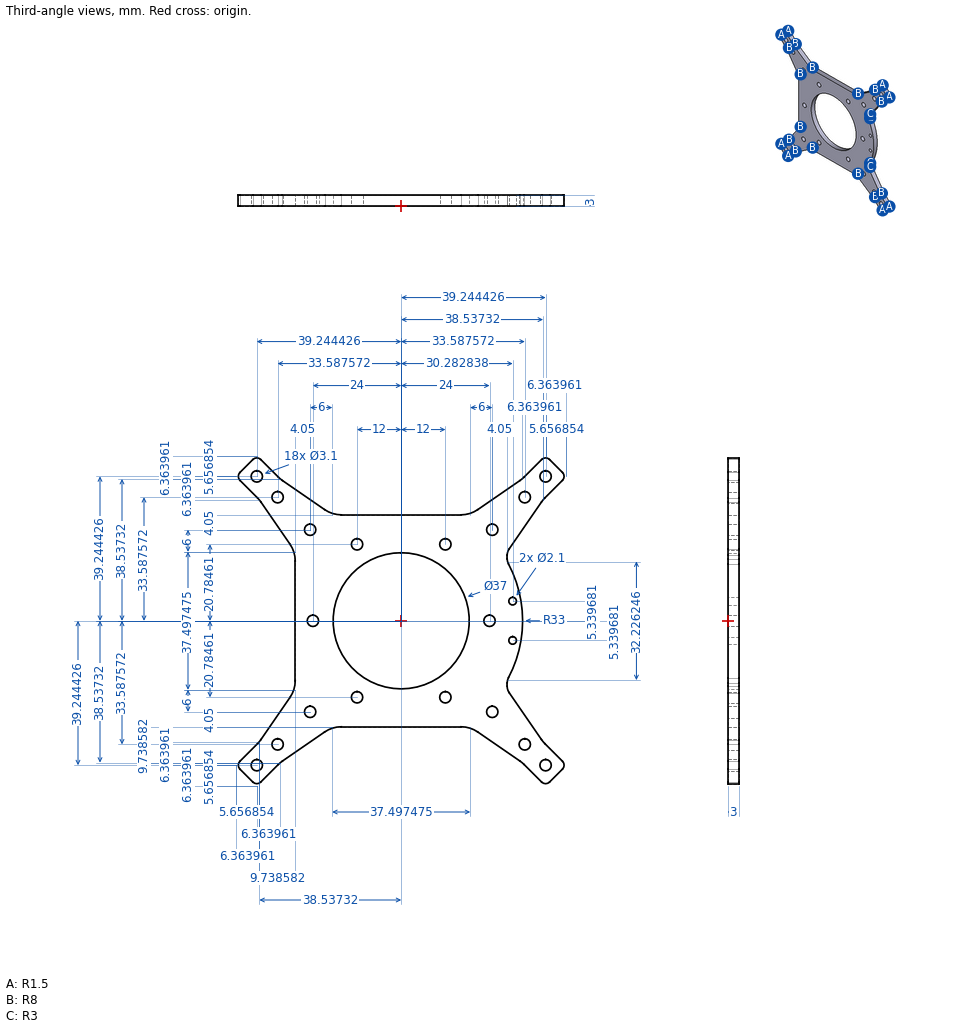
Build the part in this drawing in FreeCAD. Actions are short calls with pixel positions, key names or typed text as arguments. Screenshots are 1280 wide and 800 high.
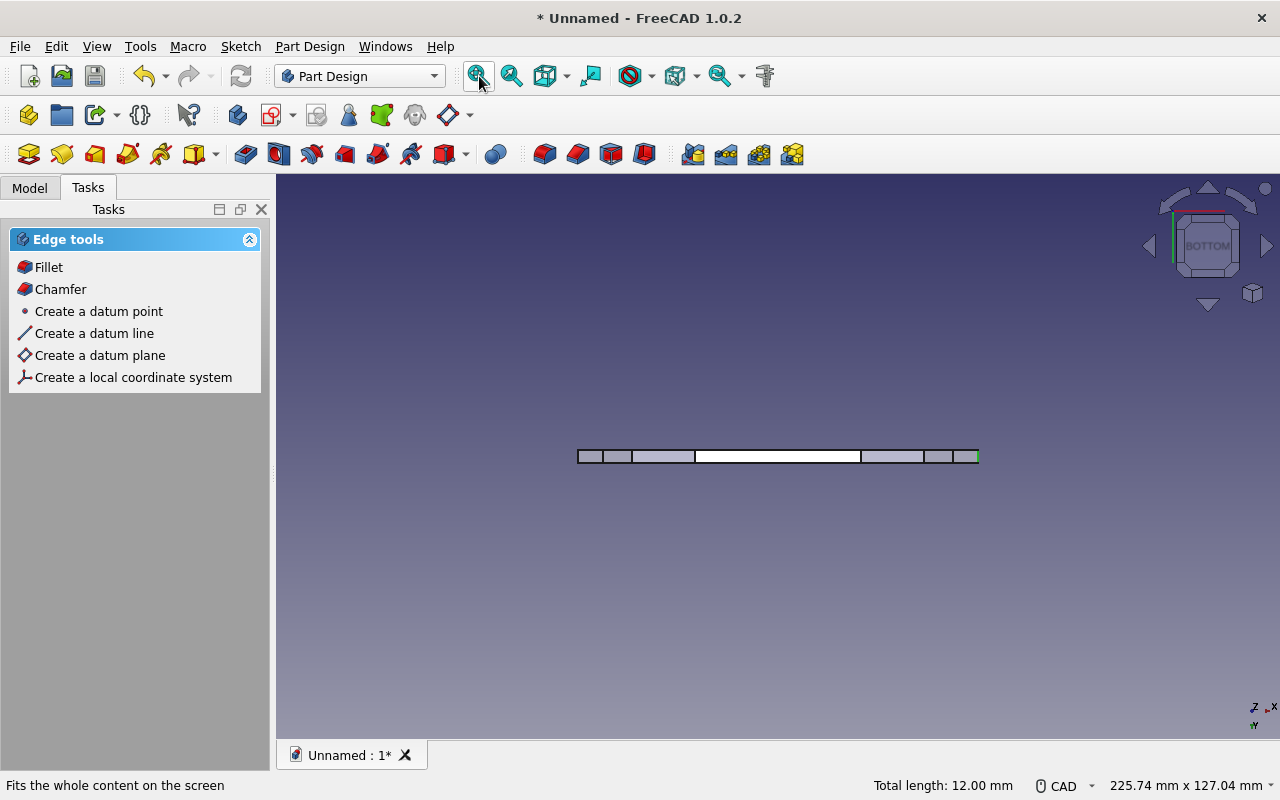
click(479, 76)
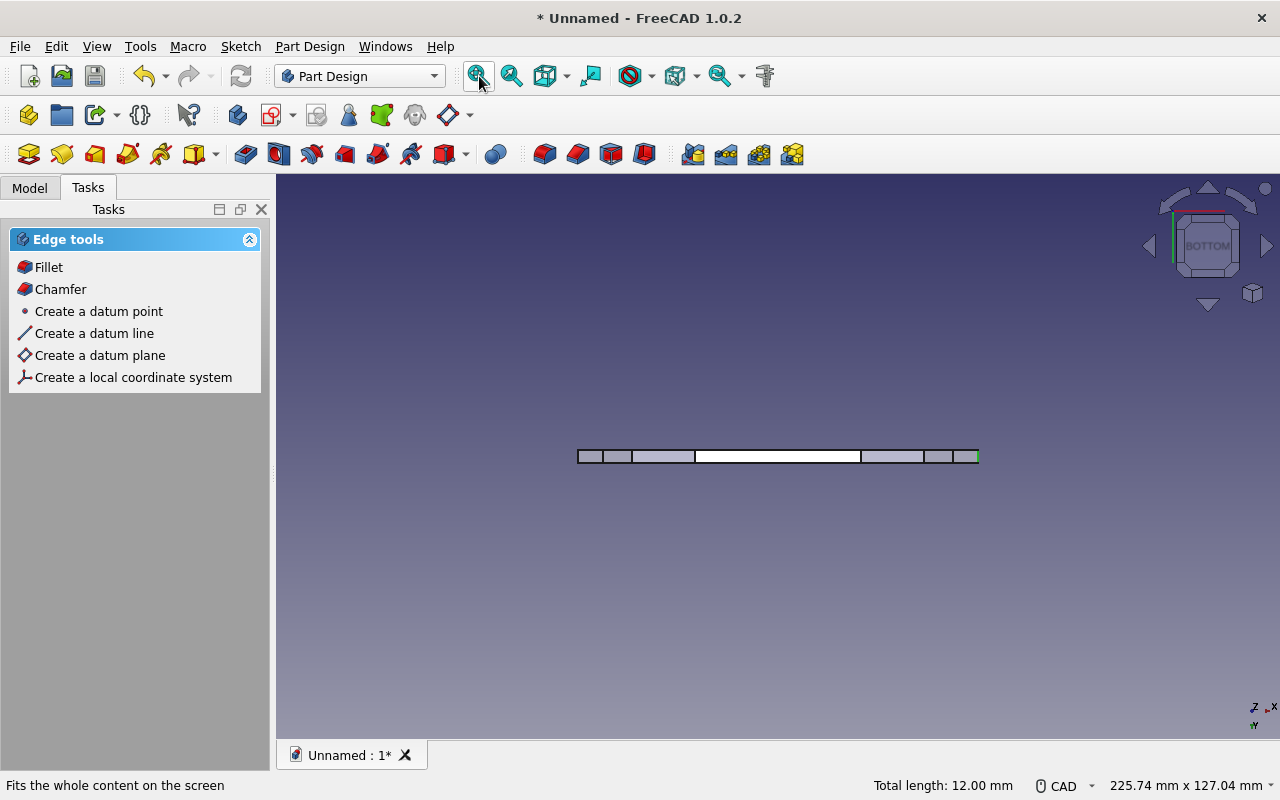
click(953, 455, ctrl)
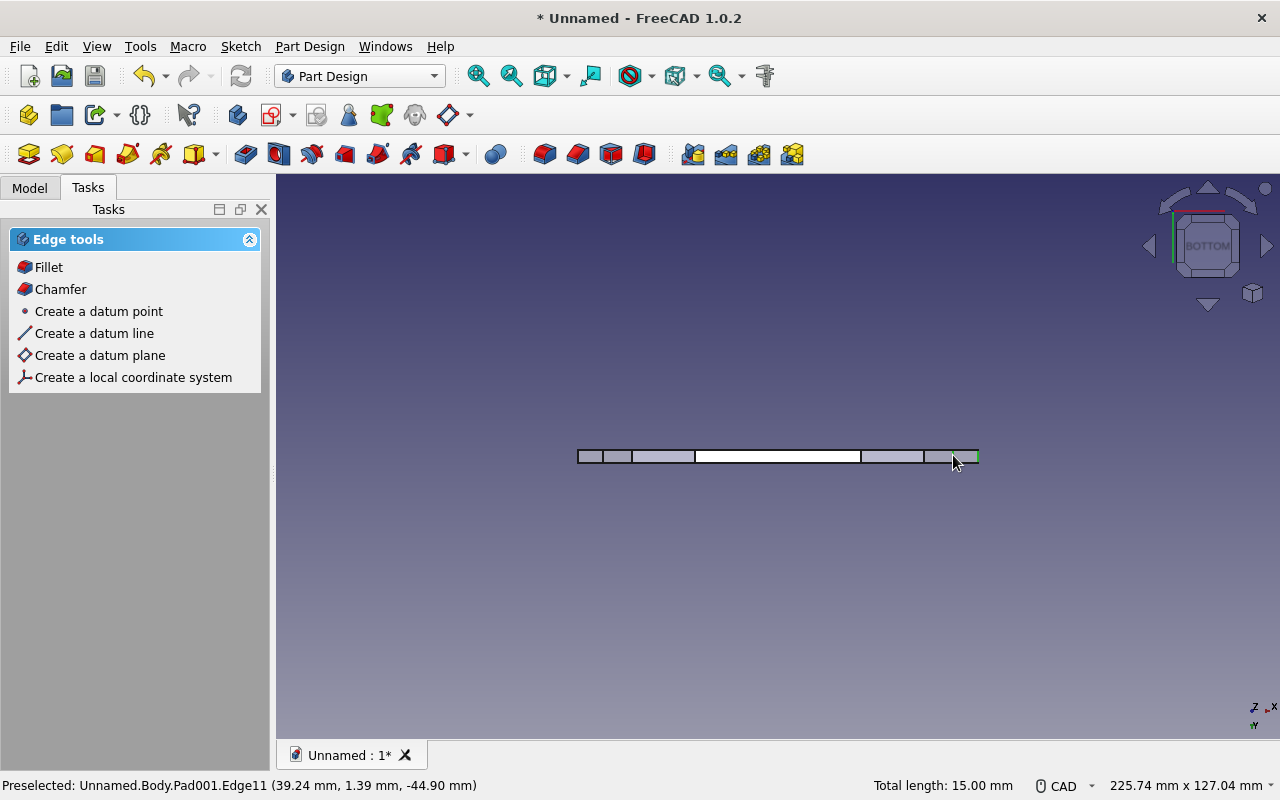
click(603, 455, ctrl)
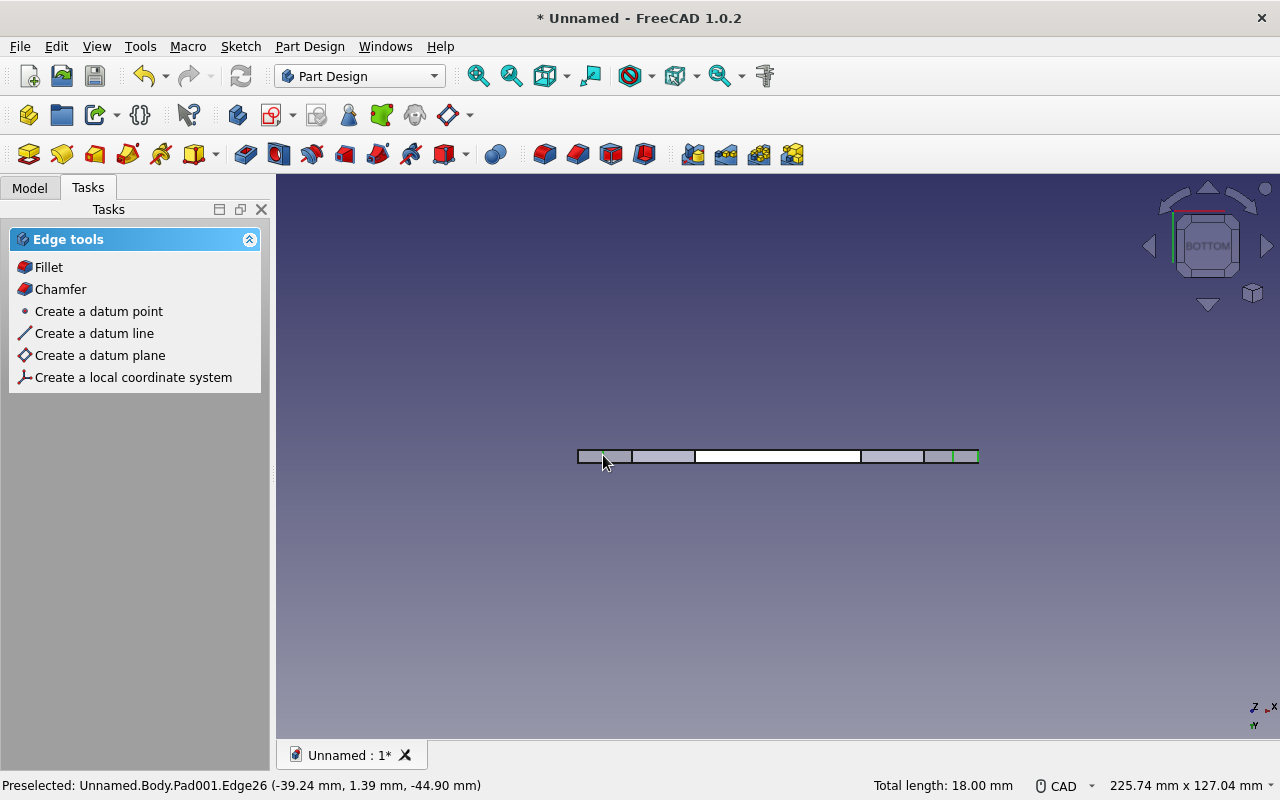
scroll(578, 455, up, 6)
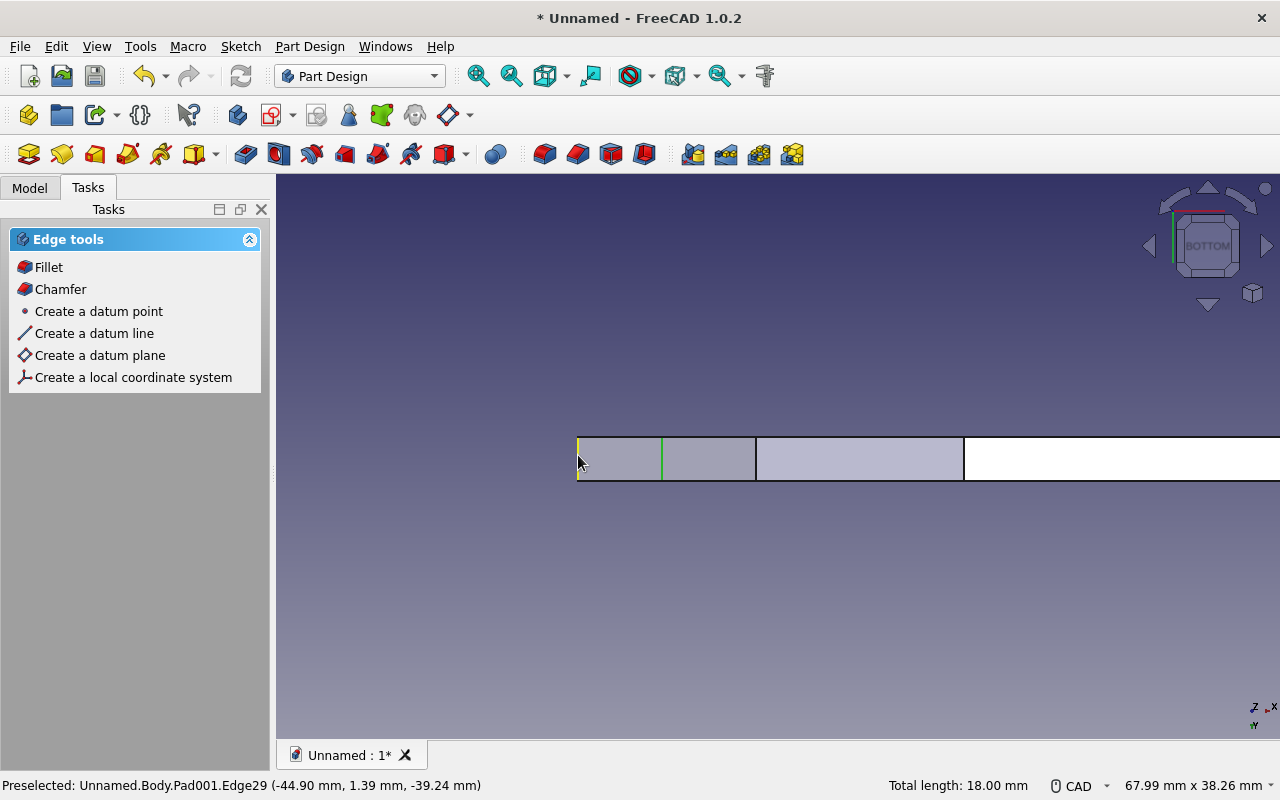
click(479, 76)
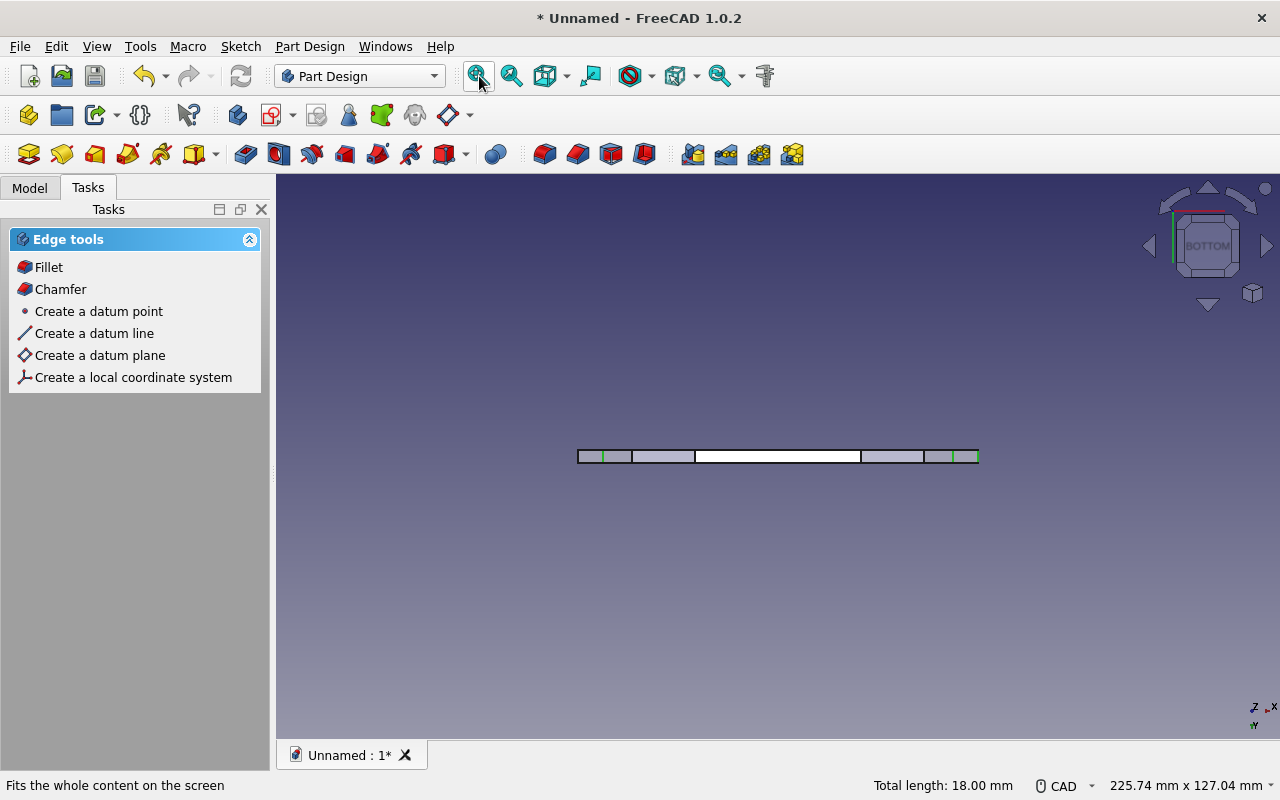
key(4)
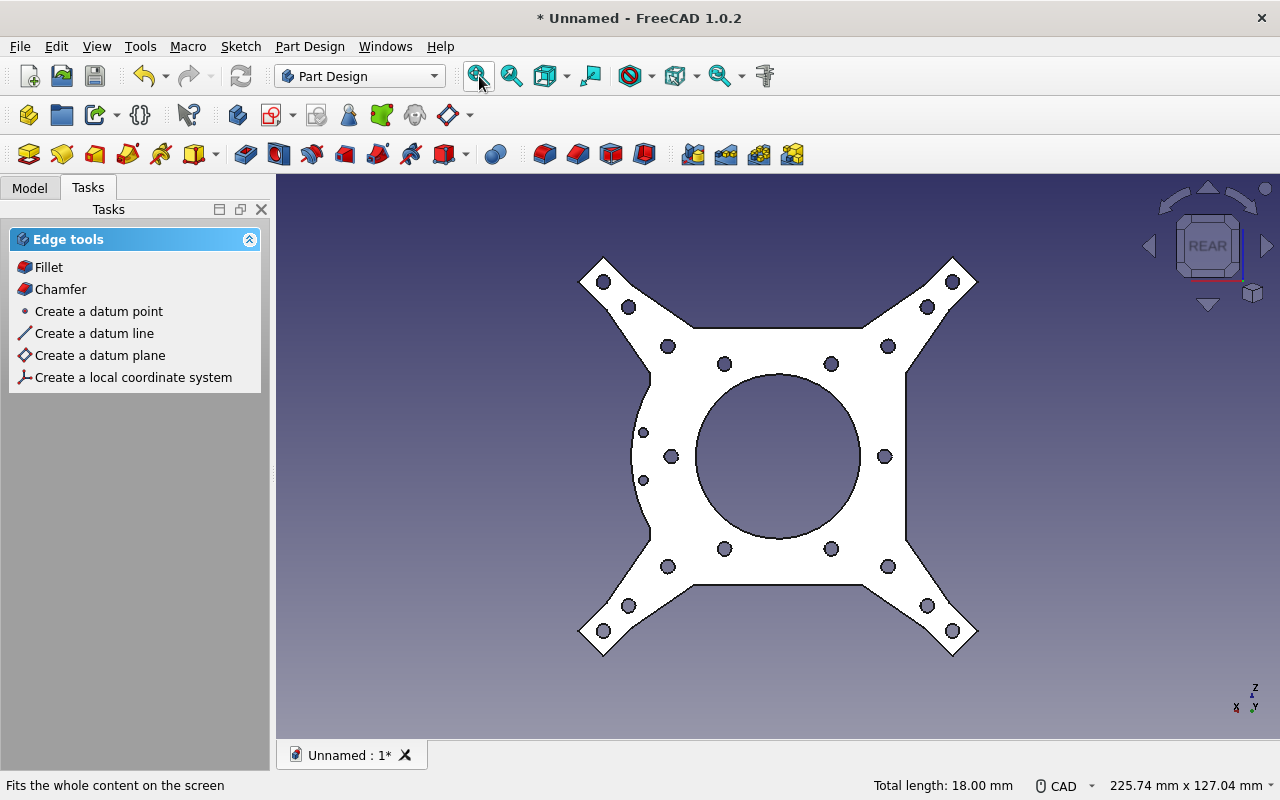
scroll(978, 281, up, 6)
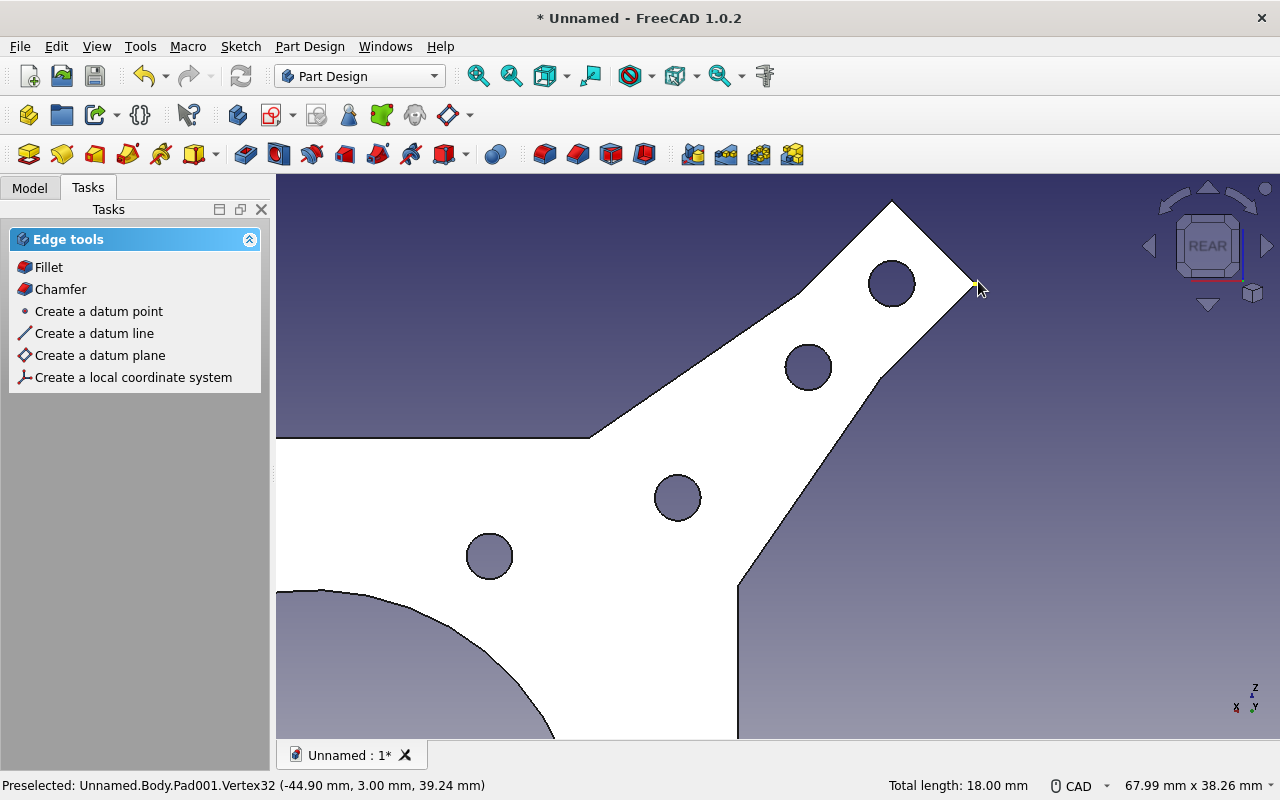
click(479, 76)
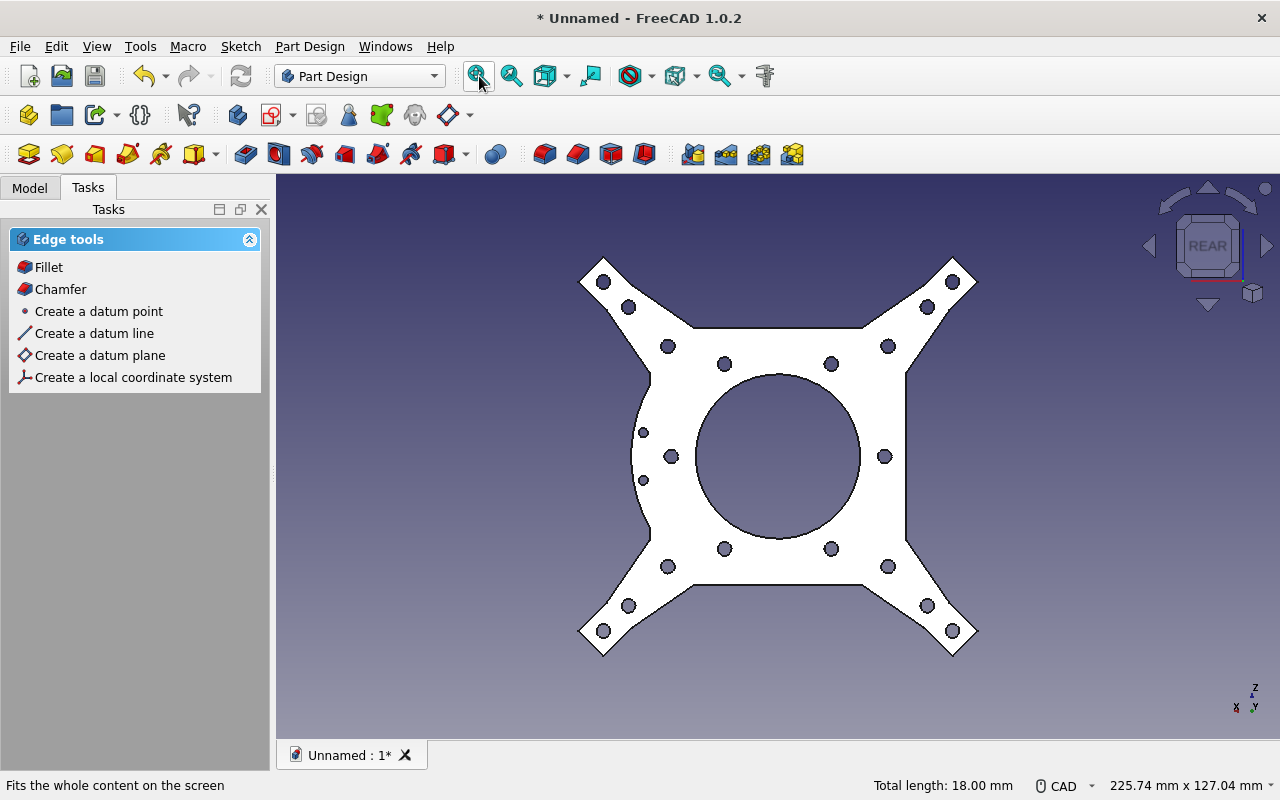
key(6)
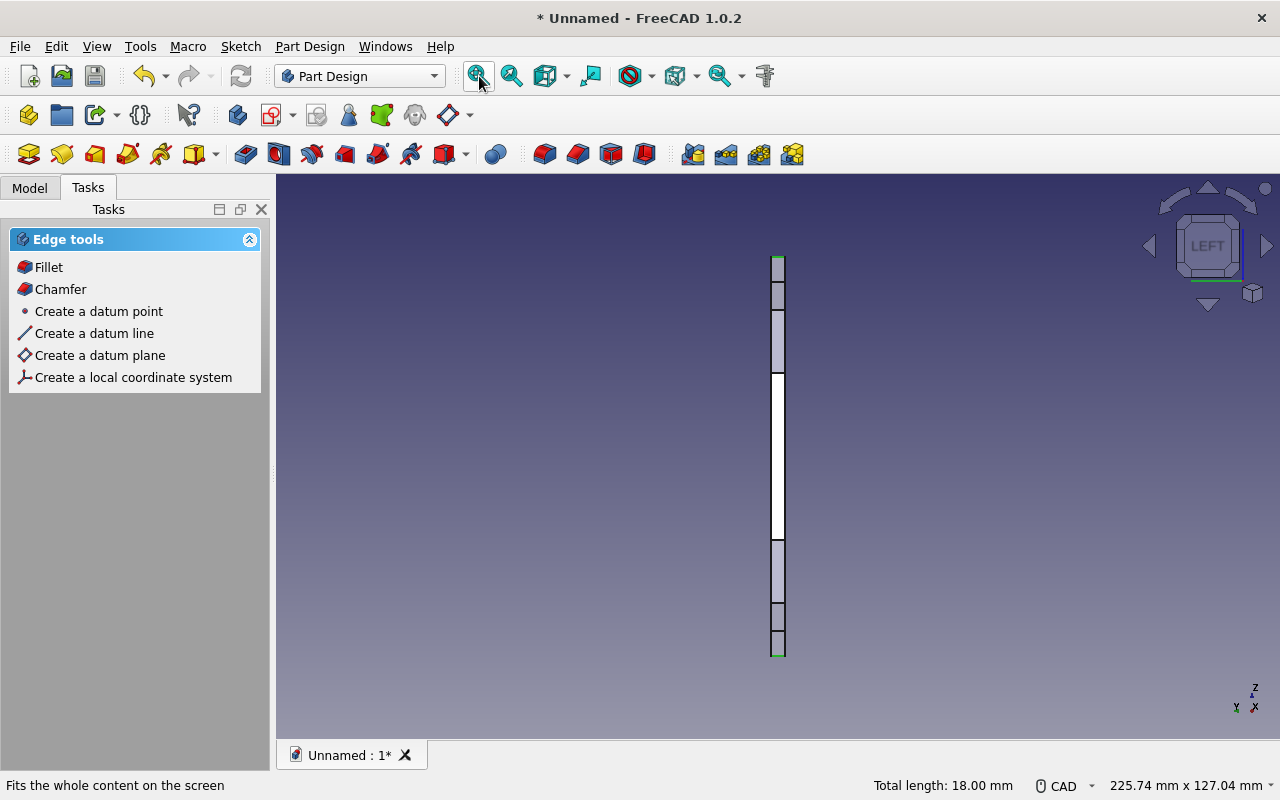
click(778, 281, ctrl)